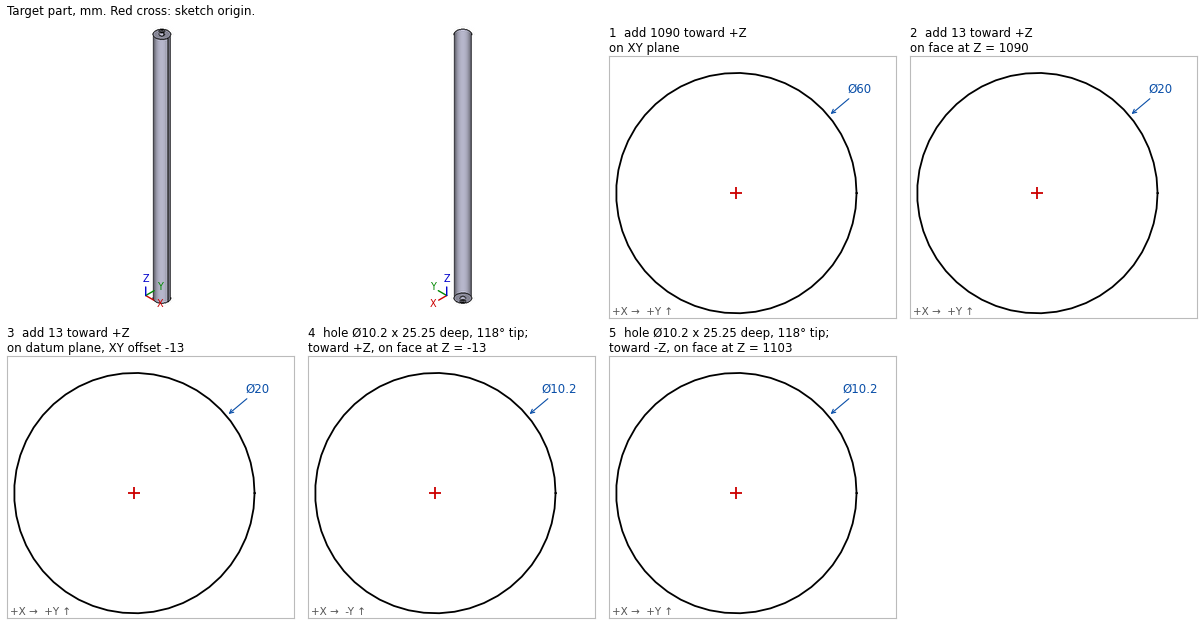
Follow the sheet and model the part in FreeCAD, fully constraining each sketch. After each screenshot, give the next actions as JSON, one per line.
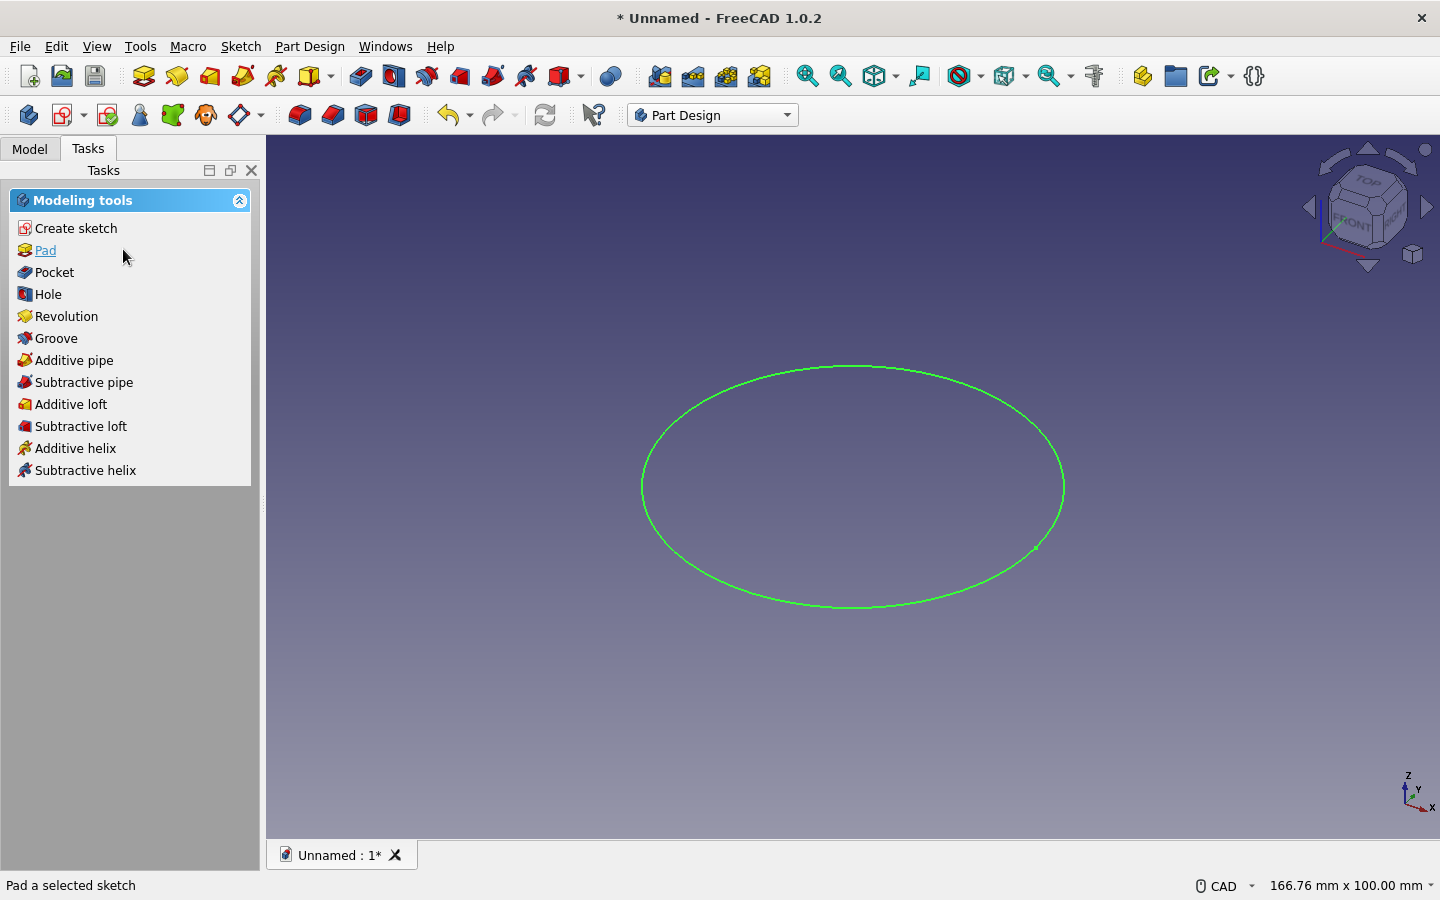
{"action": "left_click", "coordinate": [144, 76]}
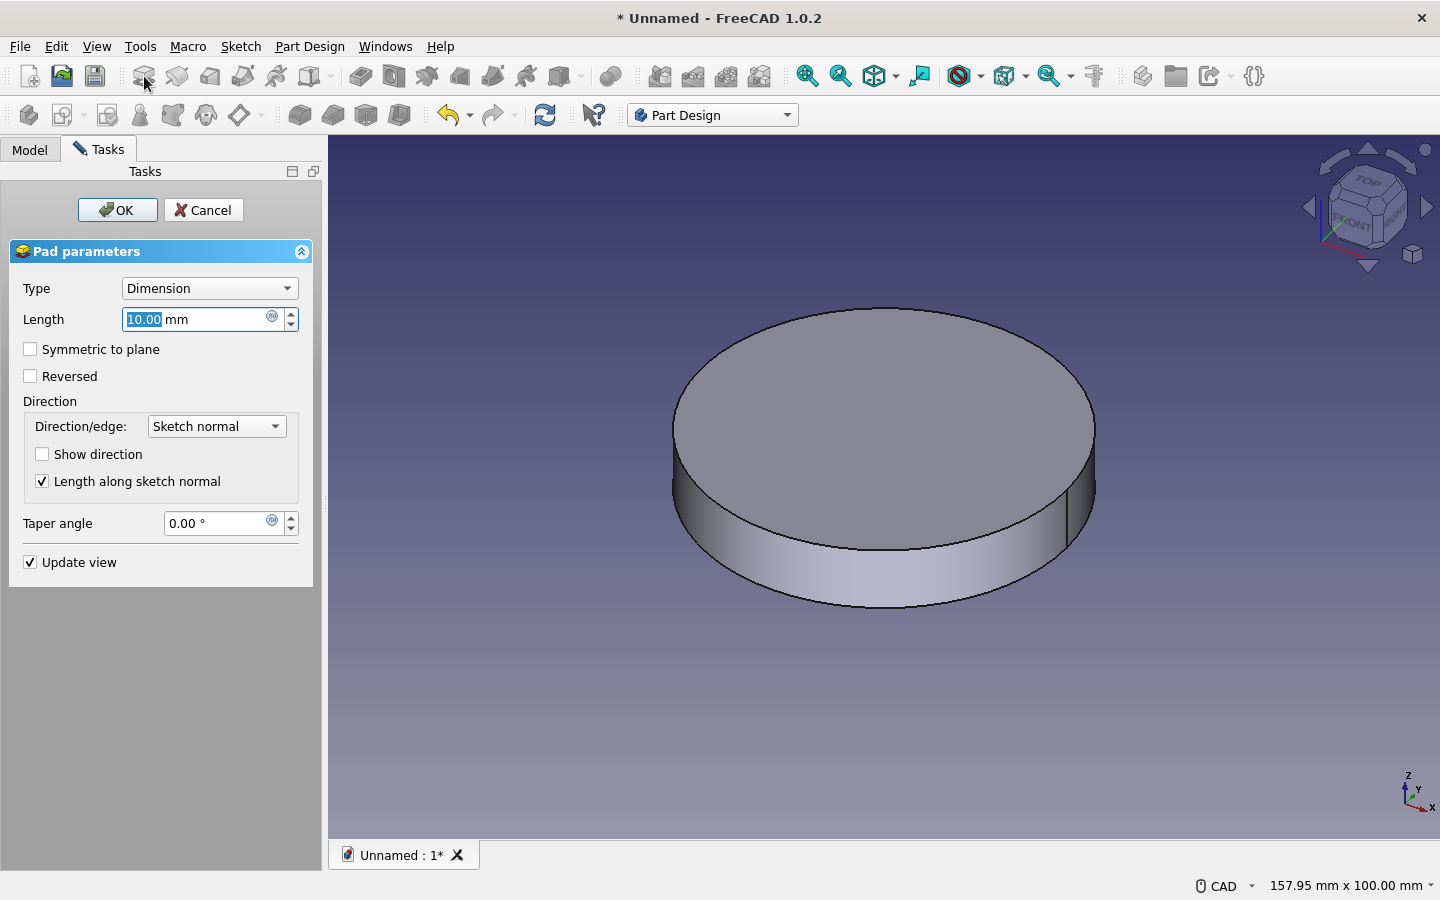
{"action": "type", "text": "1090"}
{"action": "key", "text": "Tab"}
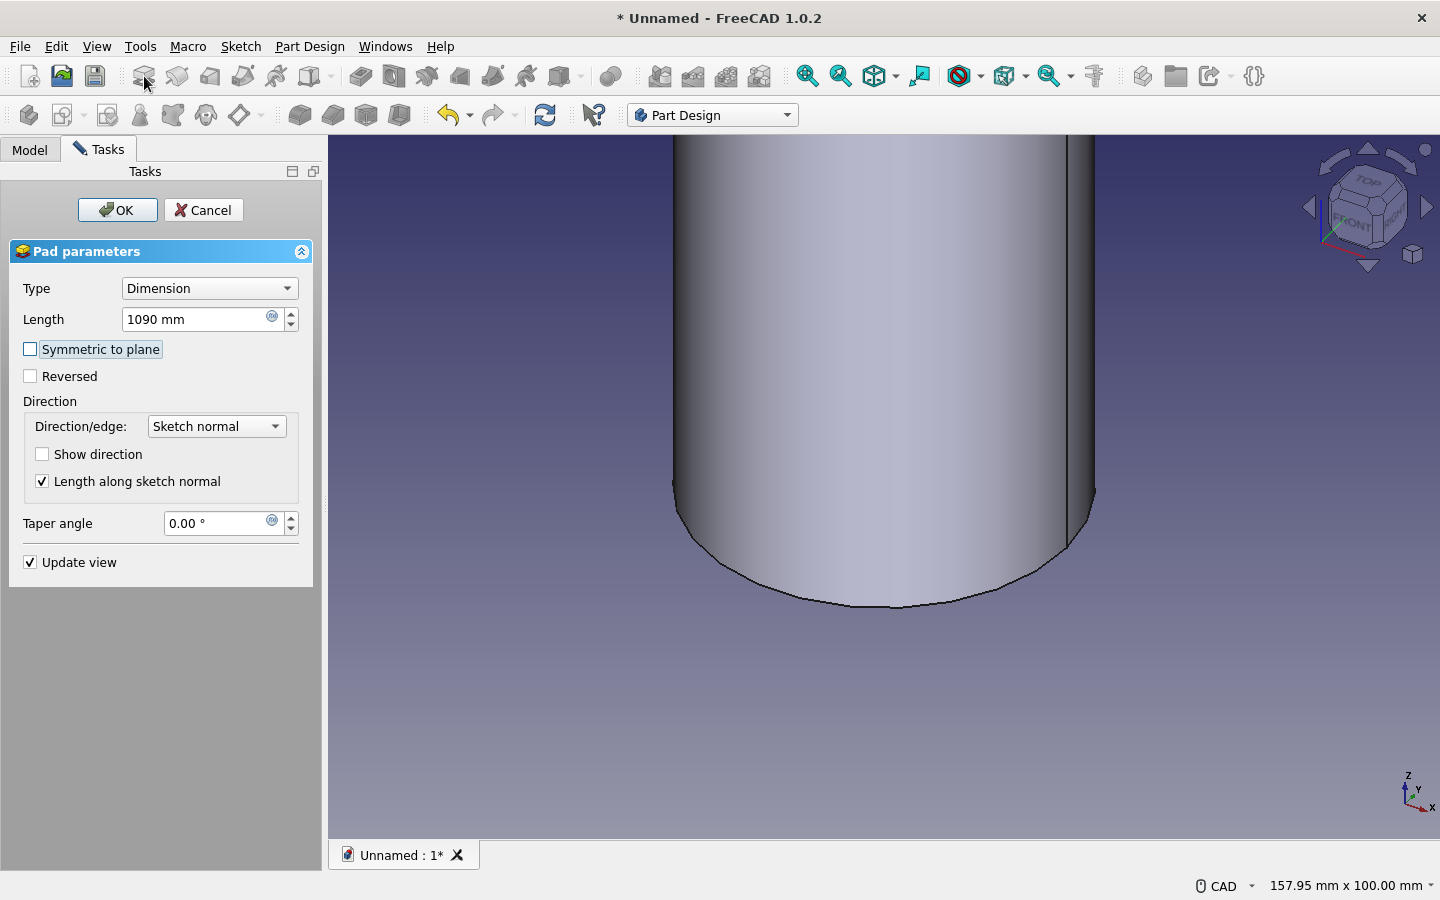
{"action": "left_click", "coordinate": [118, 210]}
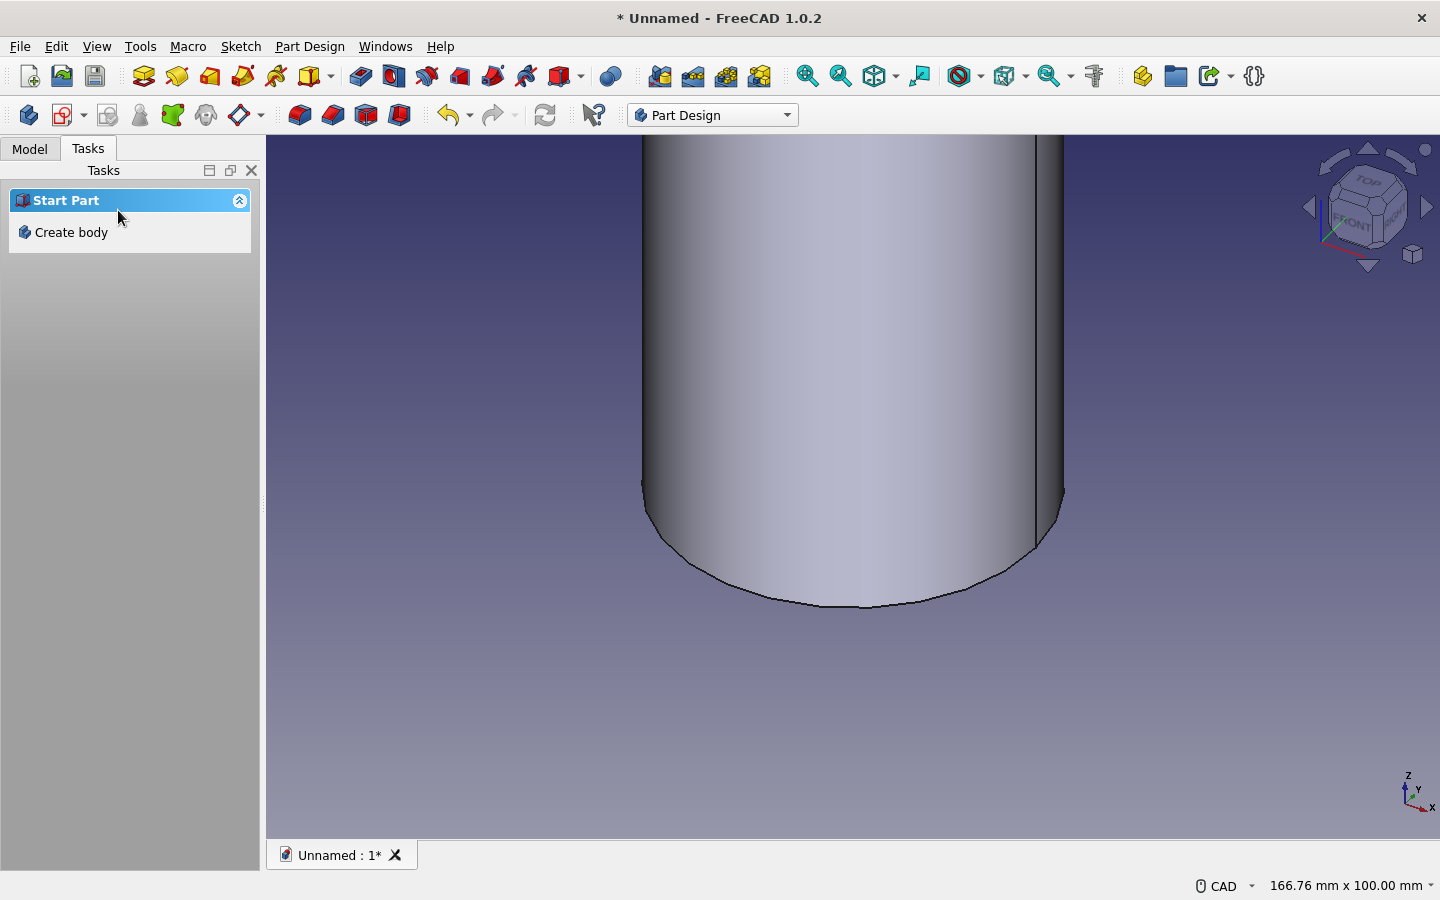
{"action": "key", "text": "v f"}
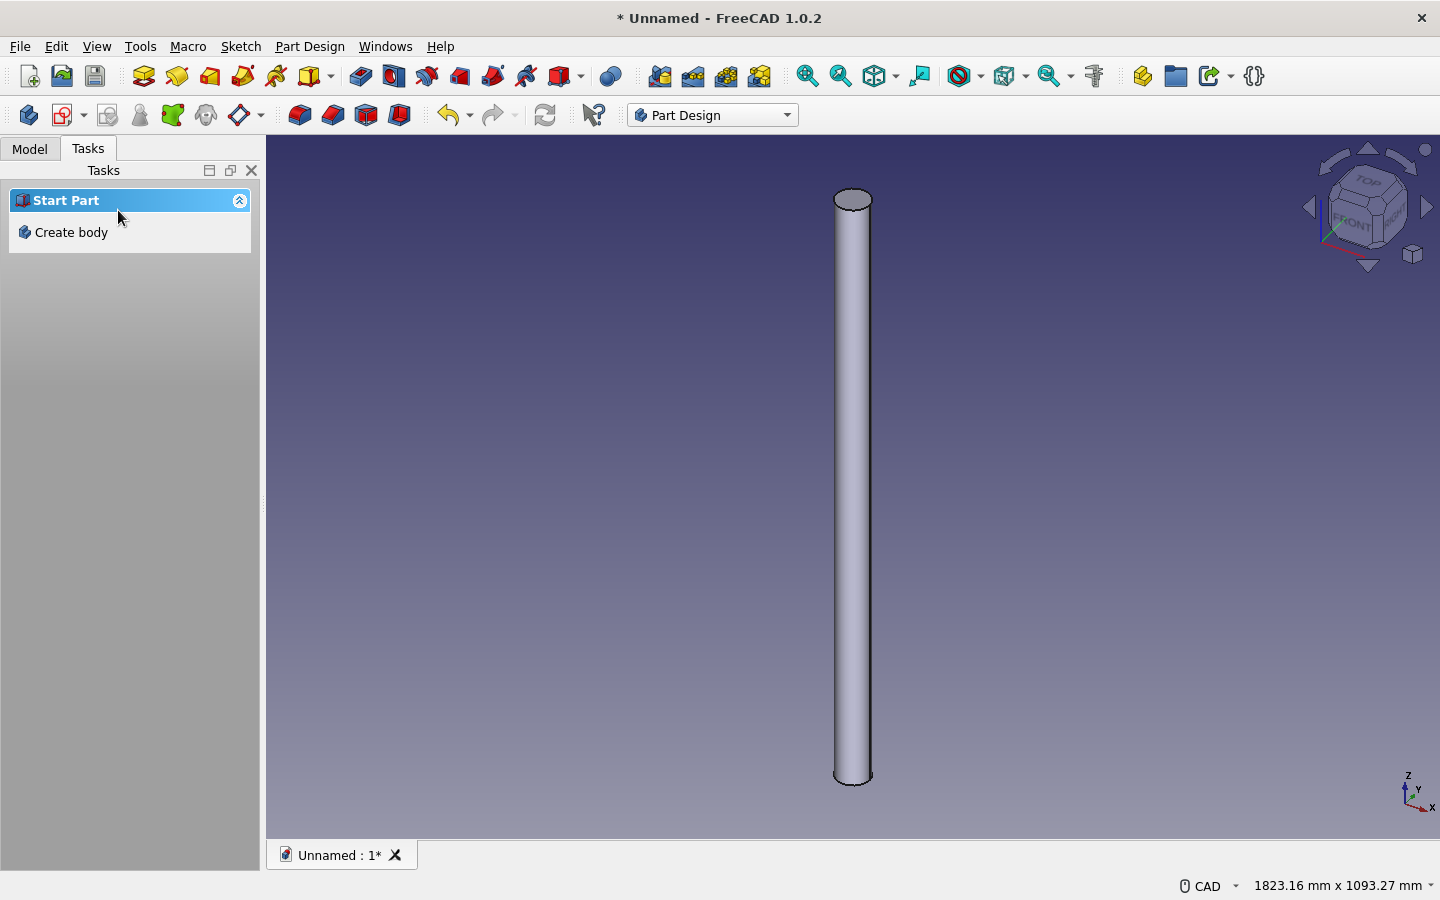
{"action": "left_click", "coordinate": [853, 199]}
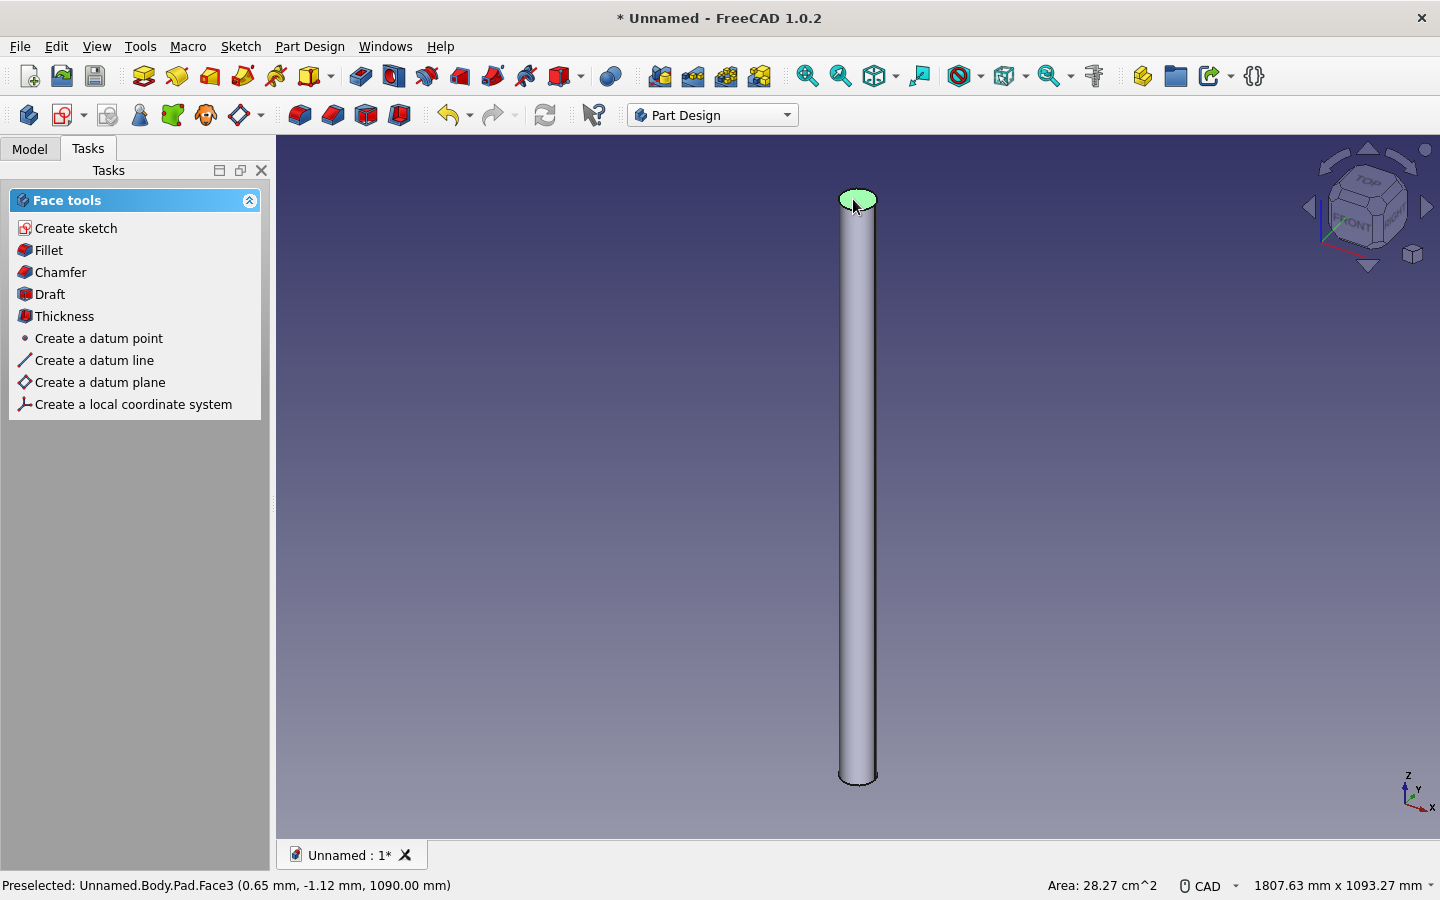
{"action": "left_click", "coordinate": [62, 116]}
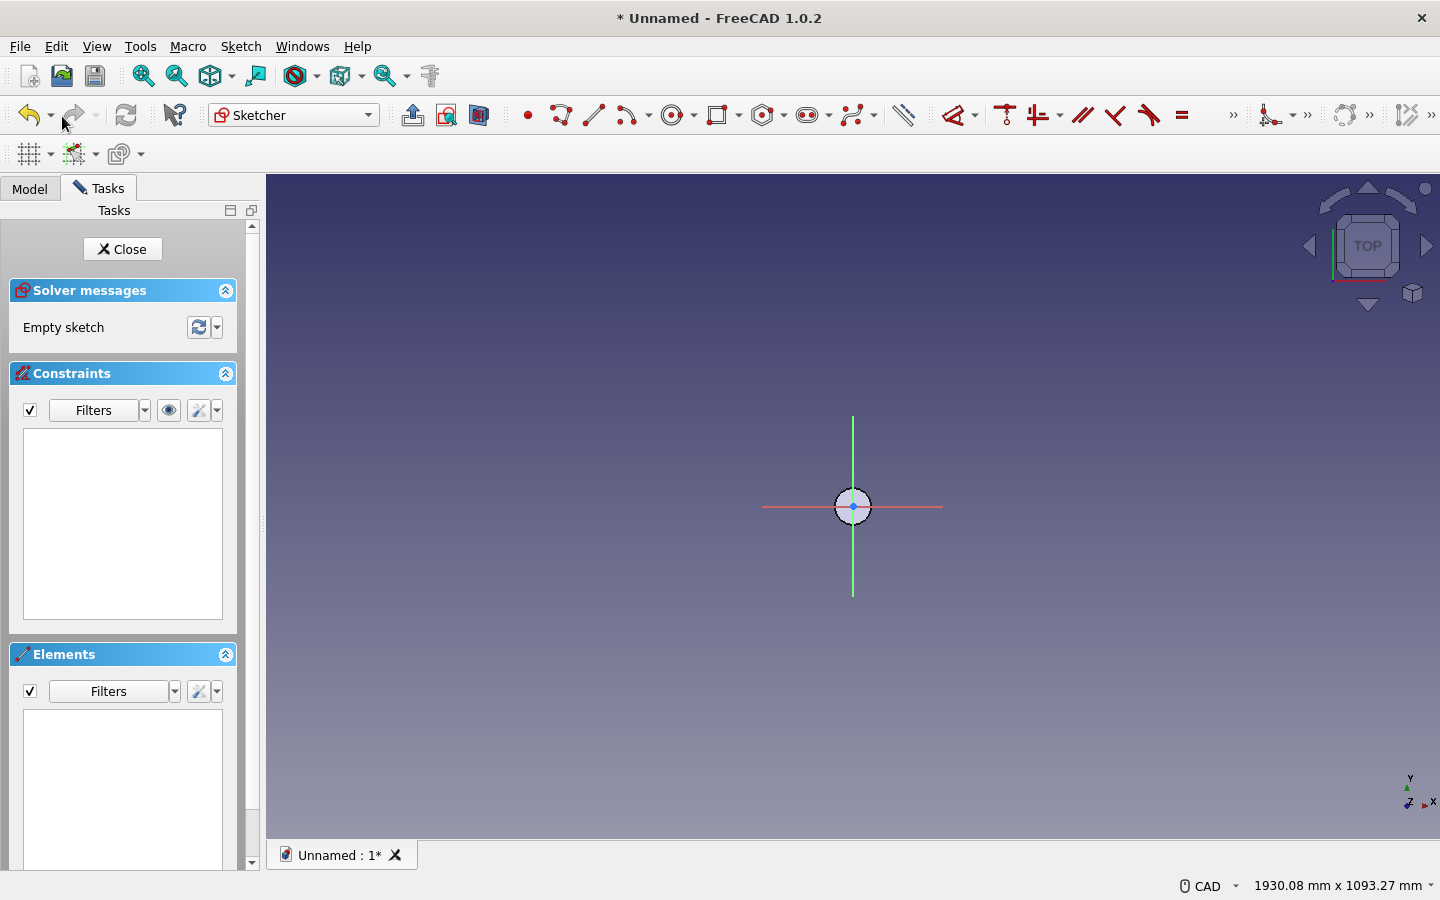
{"action": "scroll", "coordinate": [857, 506], "scroll_direction": "up", "scroll_amount": 15}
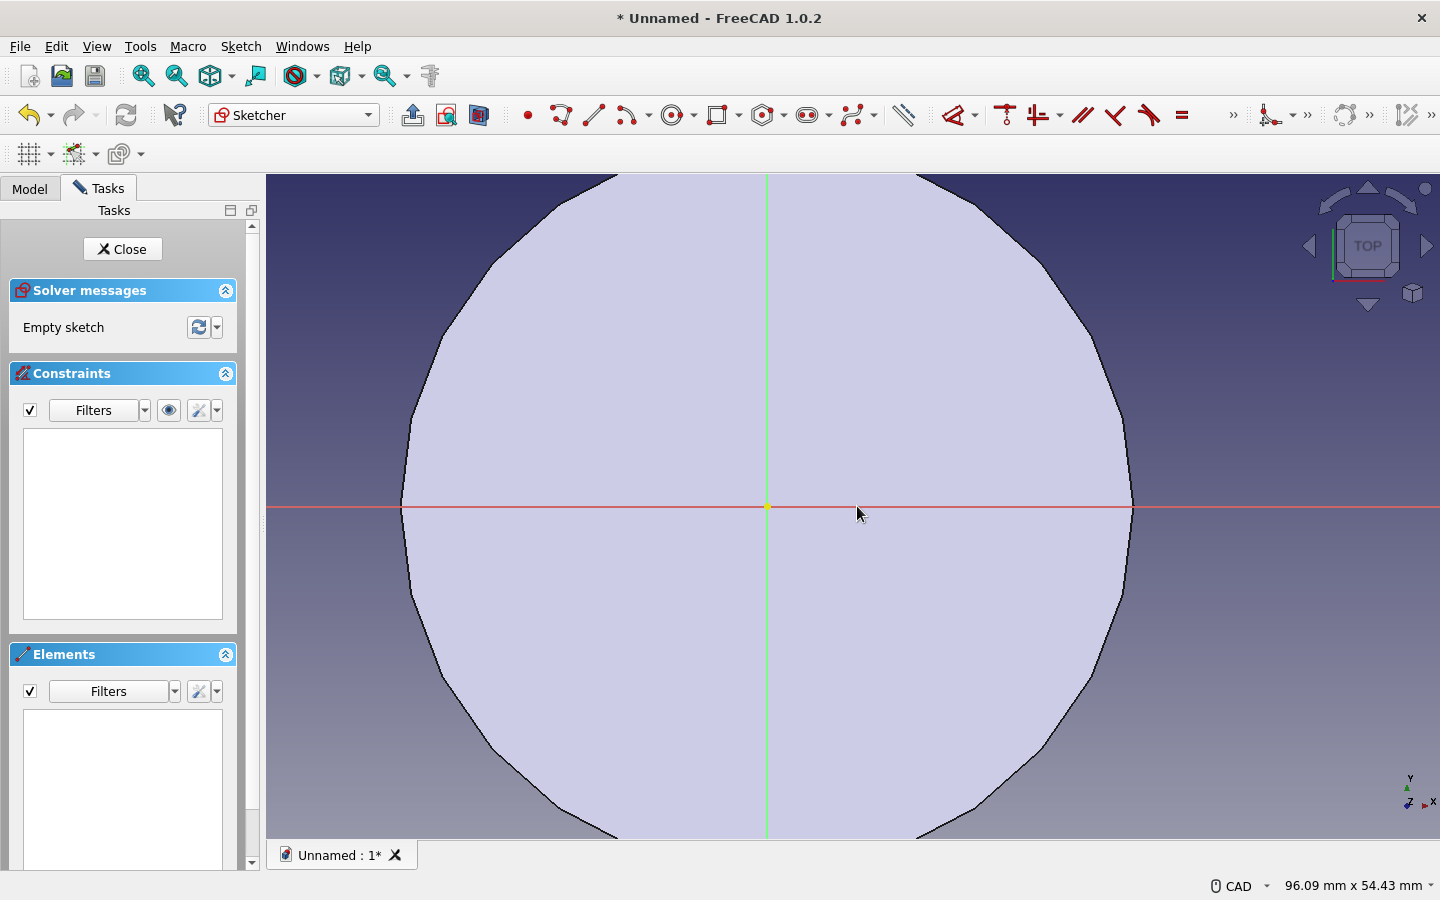
{"action": "scroll", "coordinate": [746, 507], "scroll_direction": "up", "scroll_amount": 3}